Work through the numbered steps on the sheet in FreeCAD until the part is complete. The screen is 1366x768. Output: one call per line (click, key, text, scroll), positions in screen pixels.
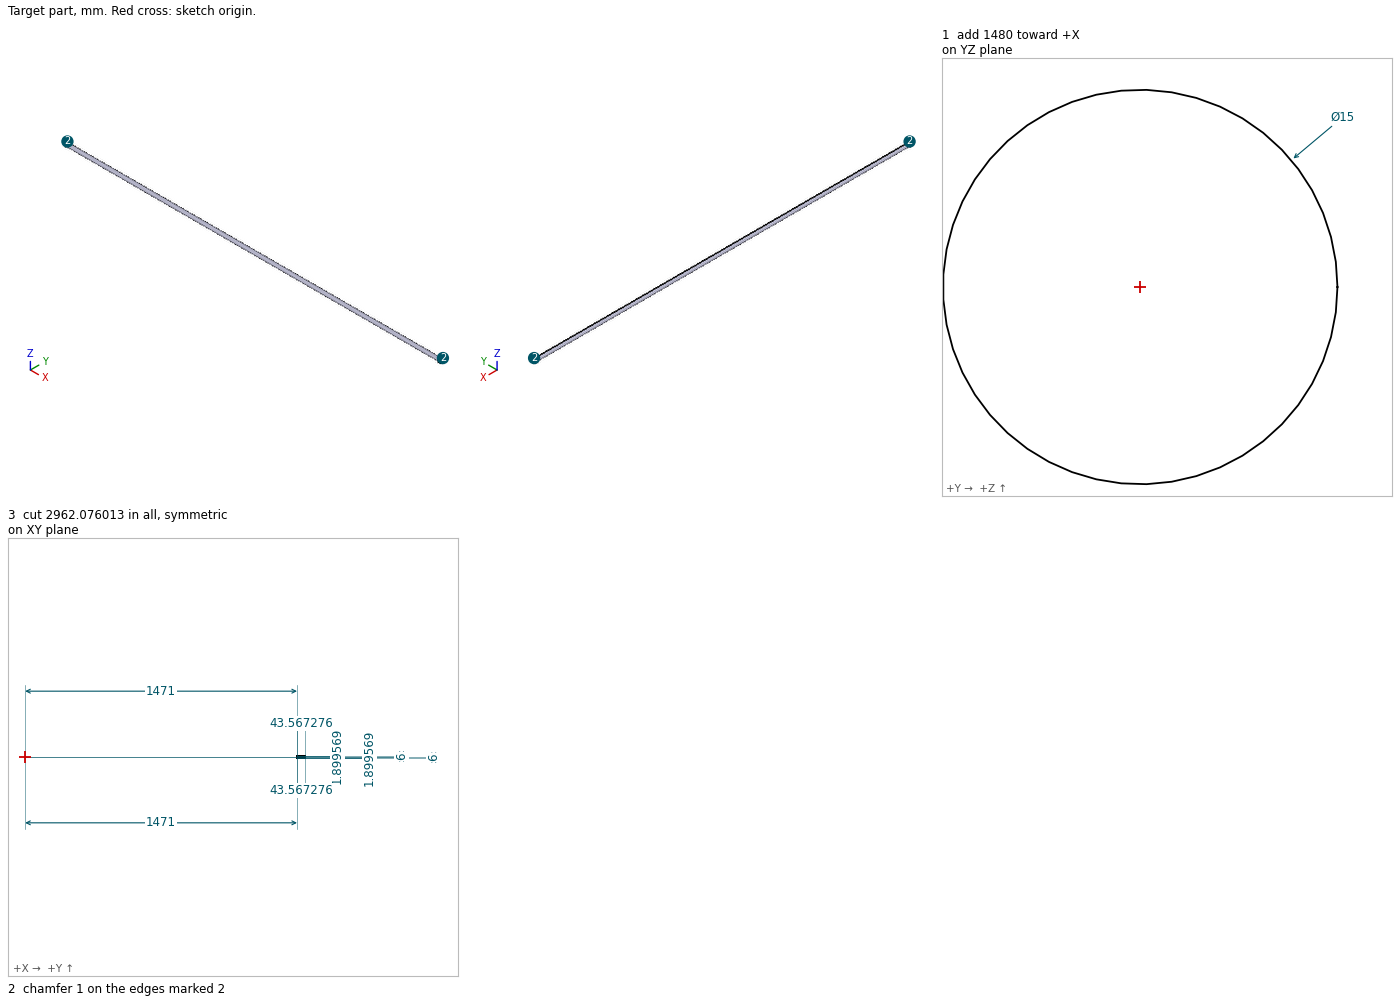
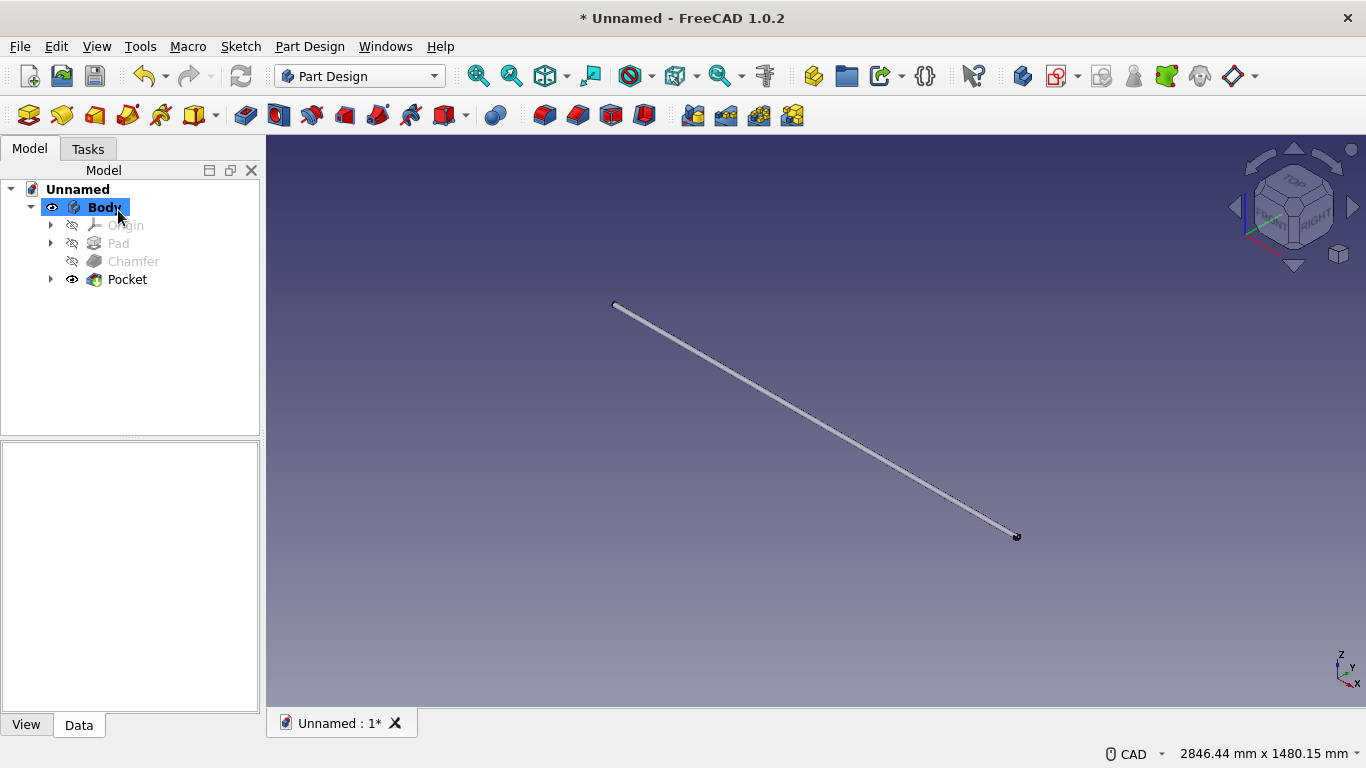
click(479, 76)